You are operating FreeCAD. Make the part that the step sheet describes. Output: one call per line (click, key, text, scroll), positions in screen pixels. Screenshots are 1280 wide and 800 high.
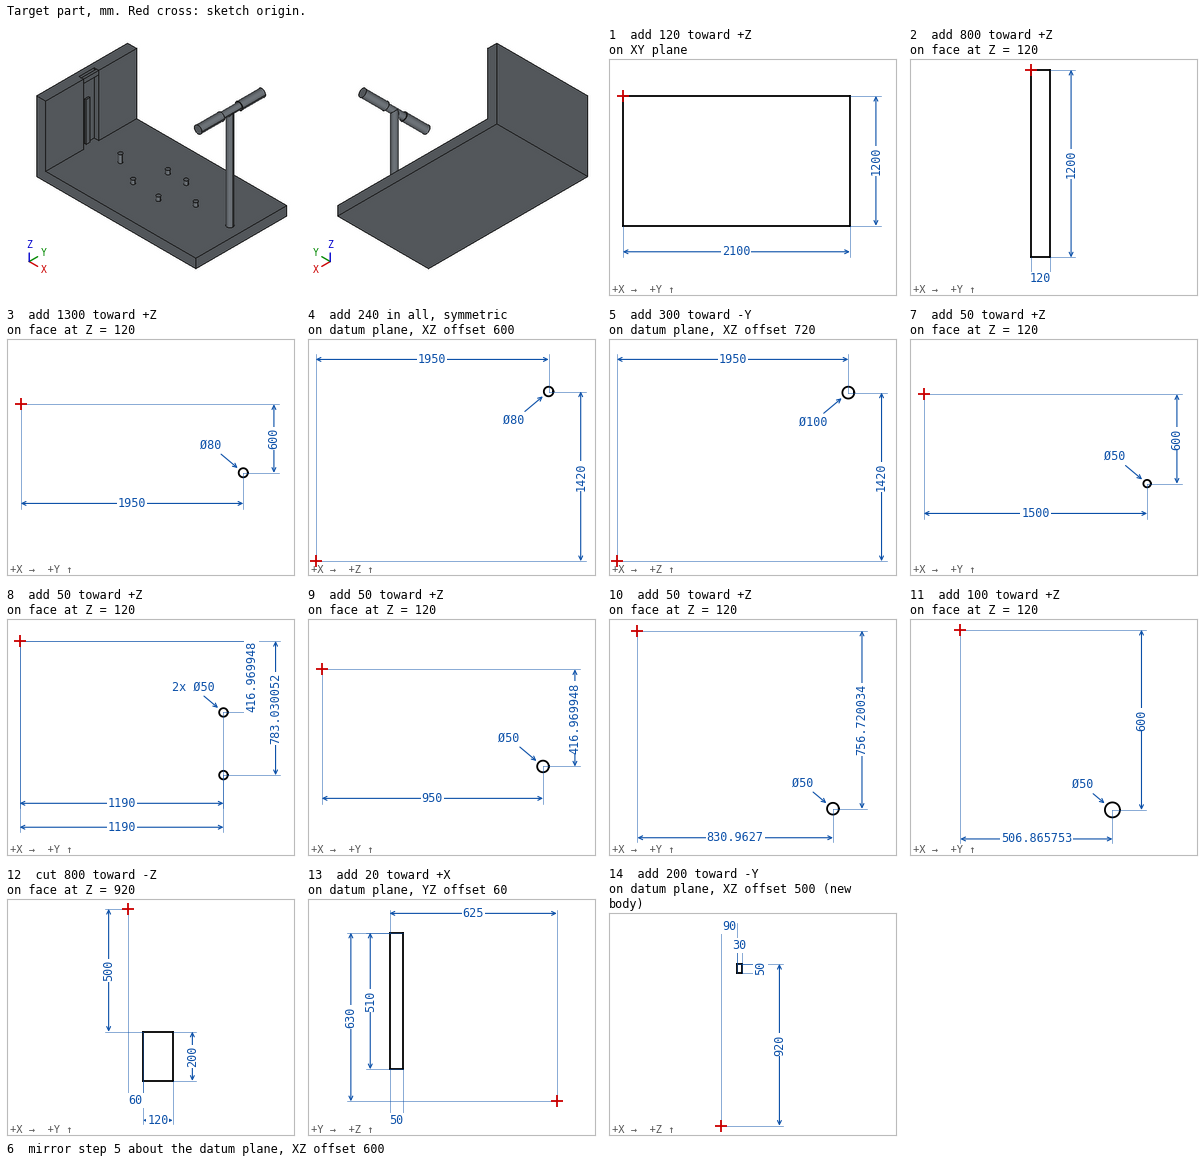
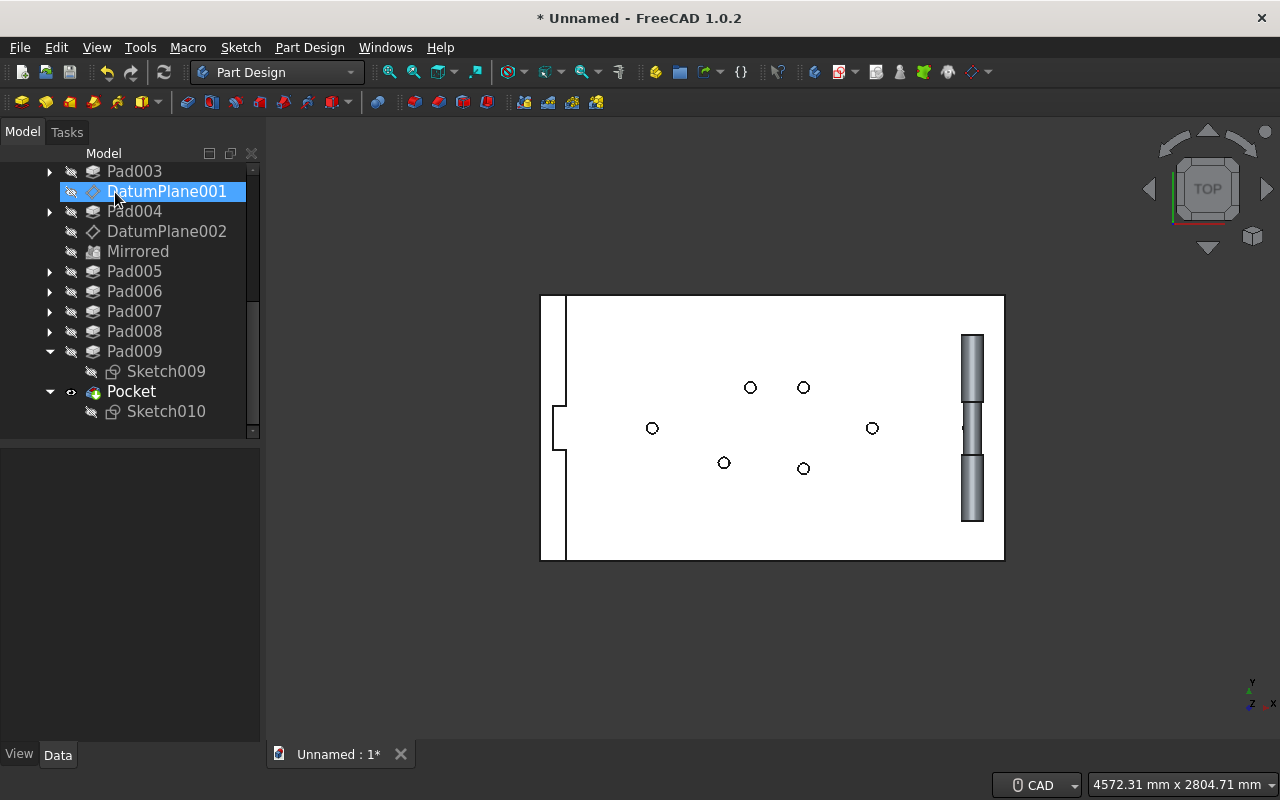
scroll(140, 287, down, 3)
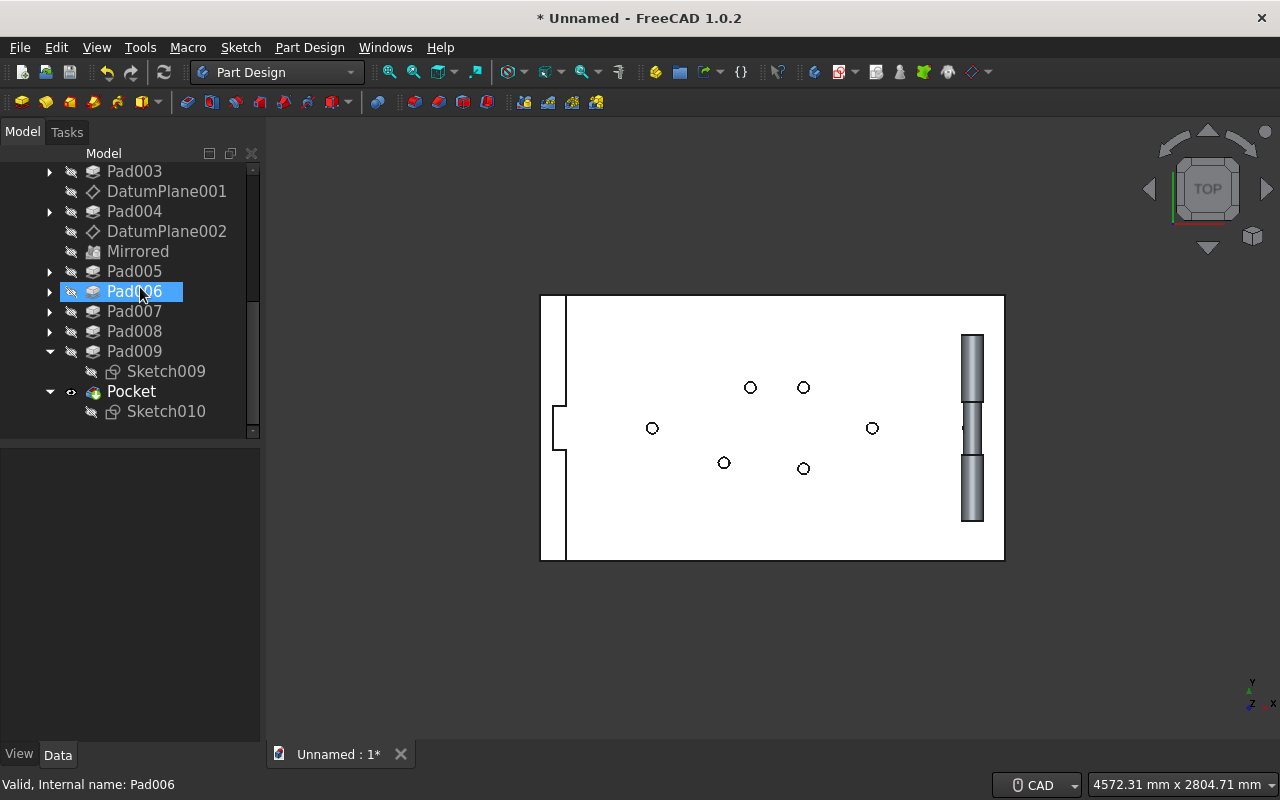
scroll(140, 287, up, 15)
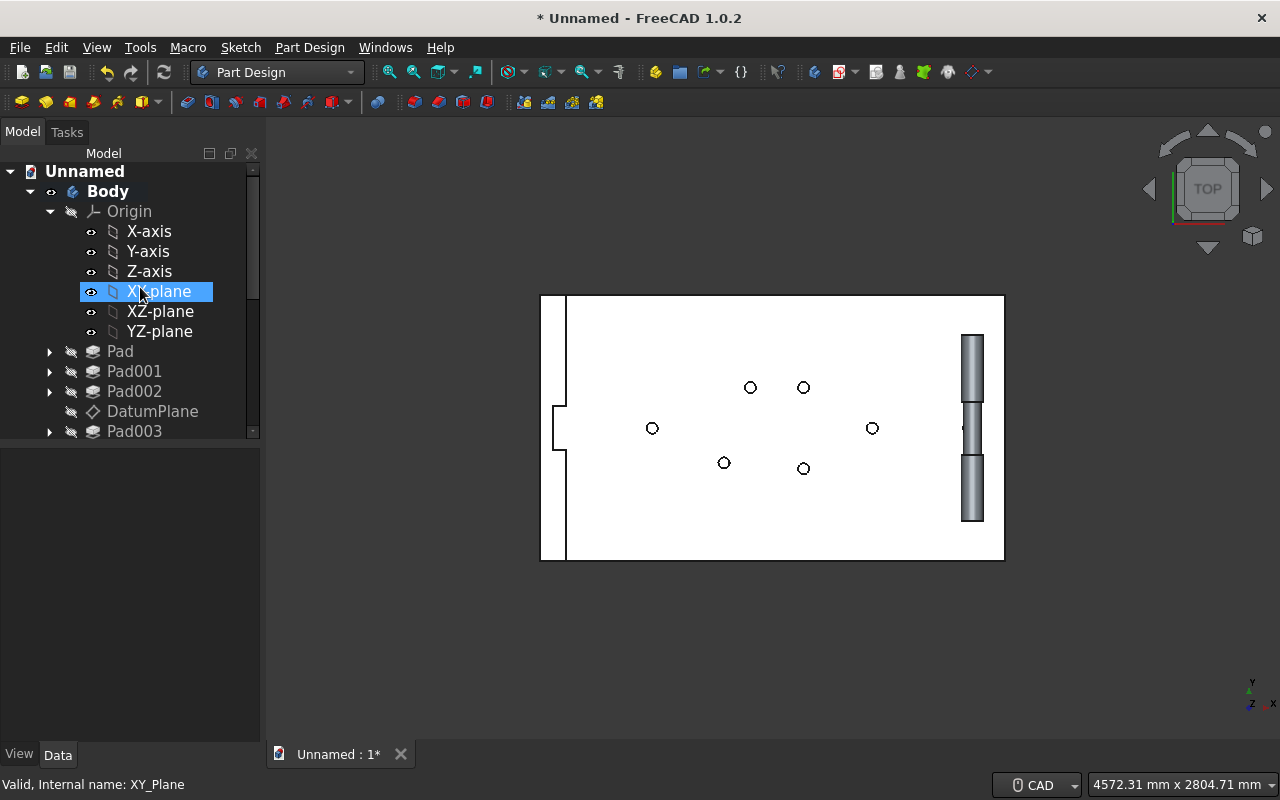
click(136, 332)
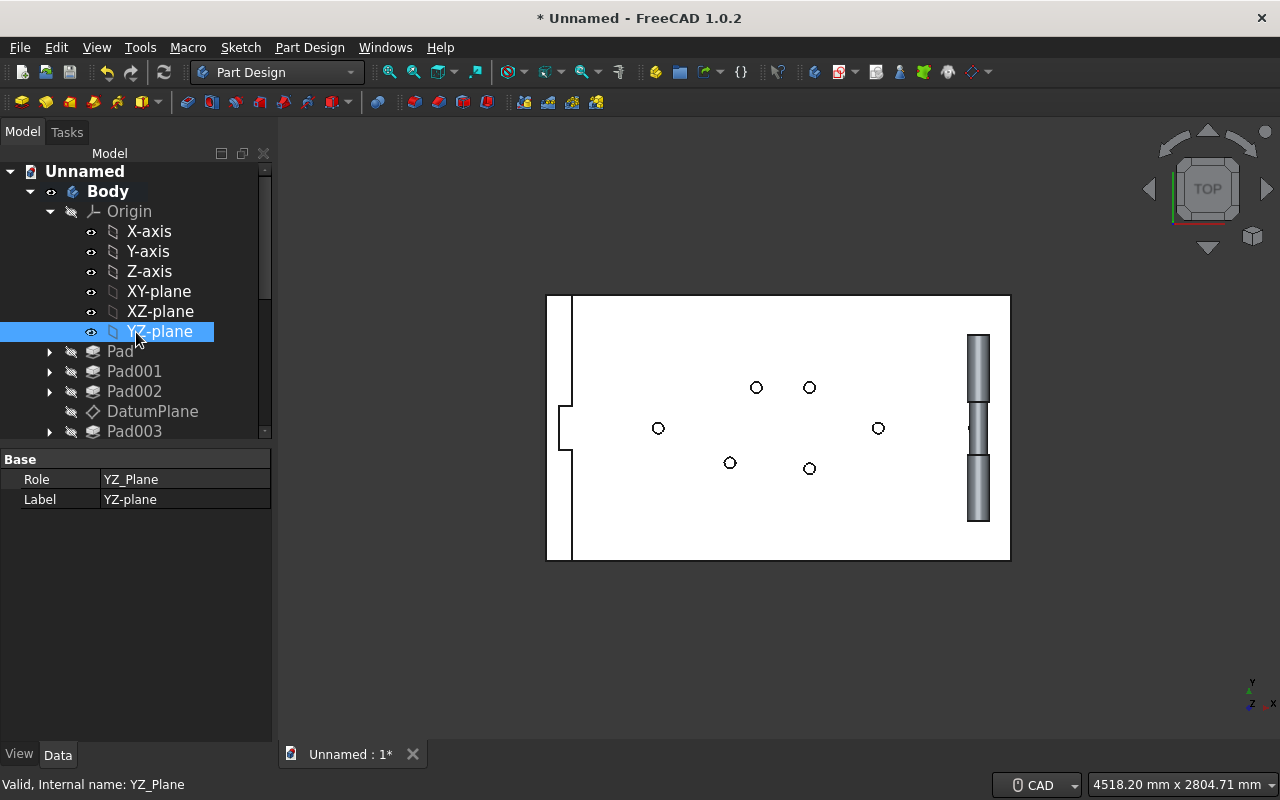
click(972, 72)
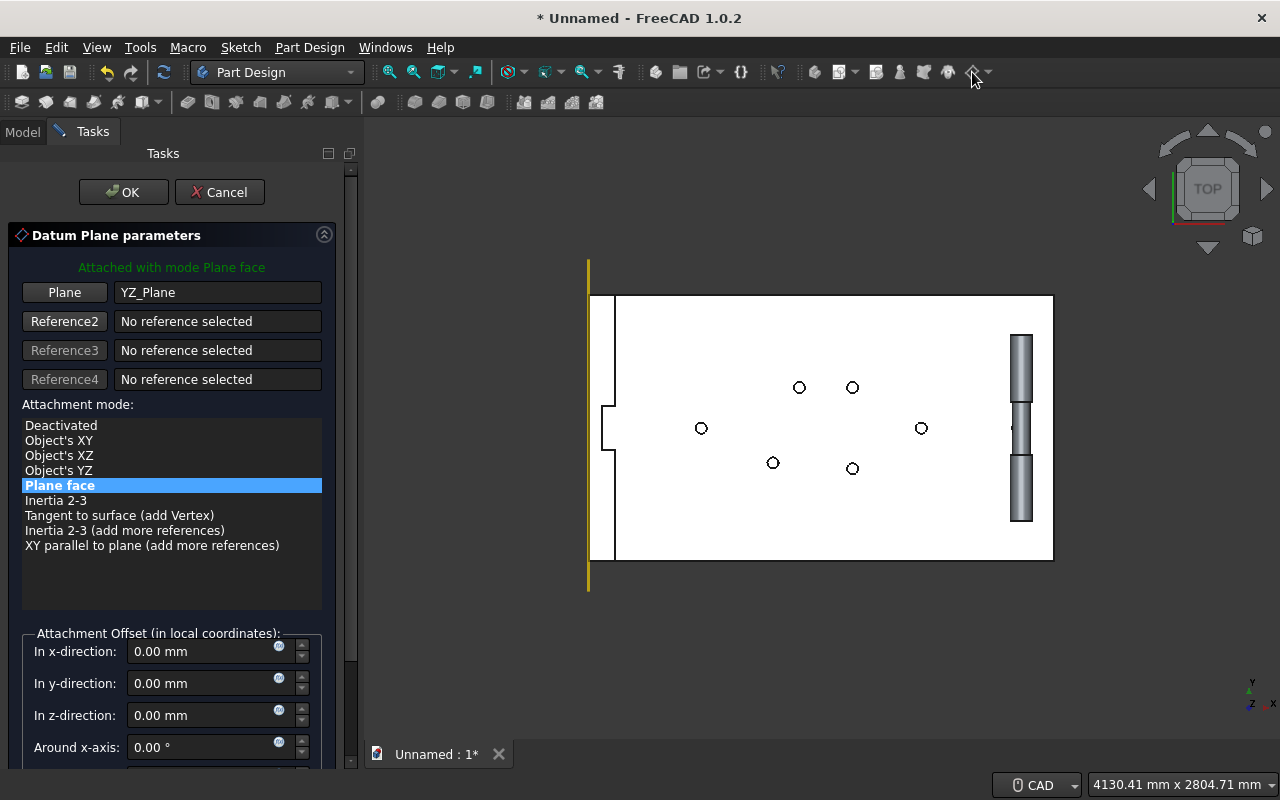
triple_click(210, 715)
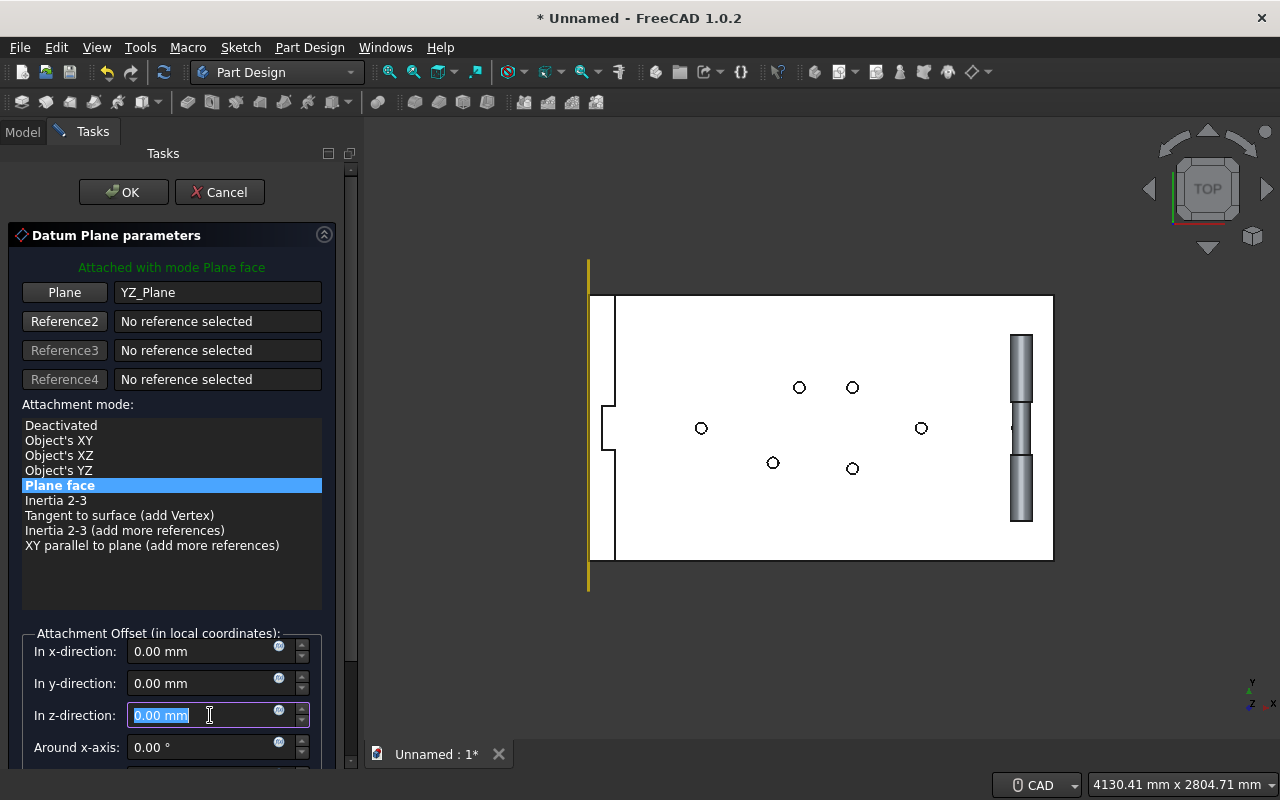
text(60)
key(Tab)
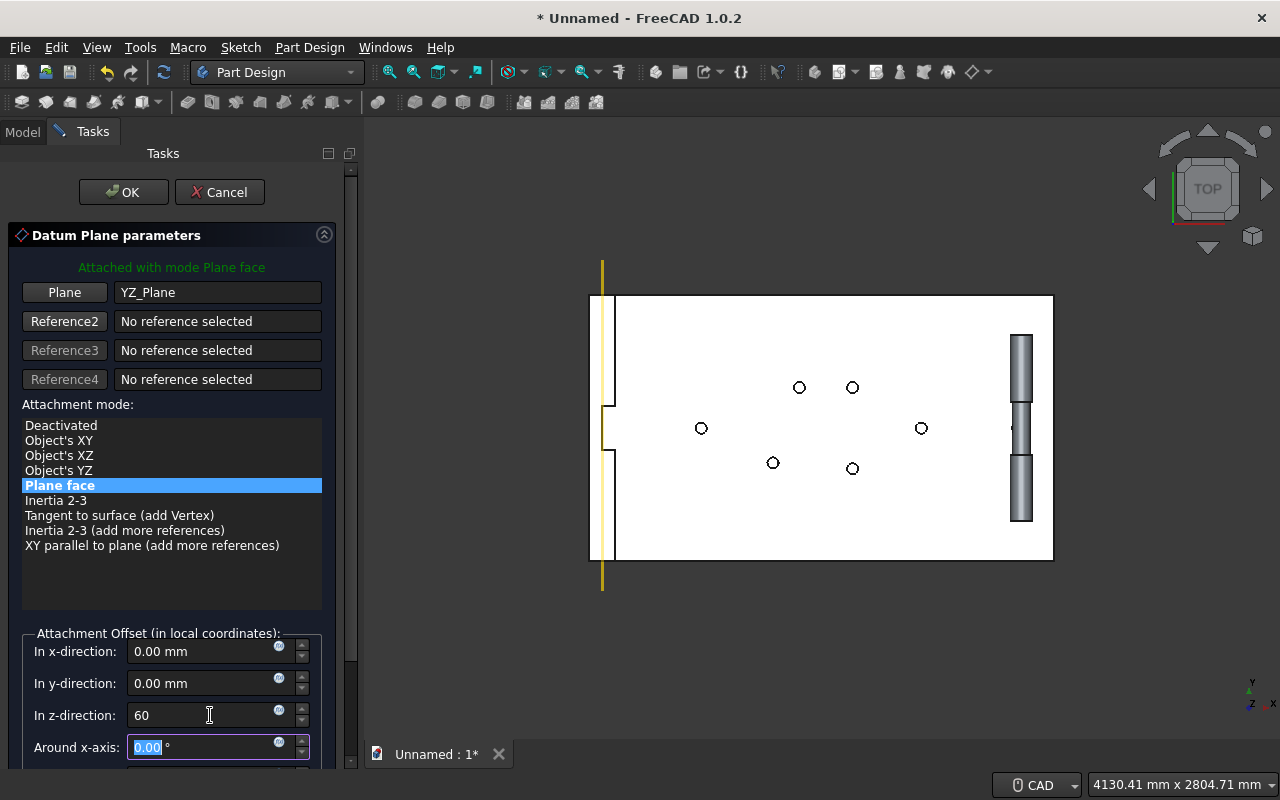
click(124, 192)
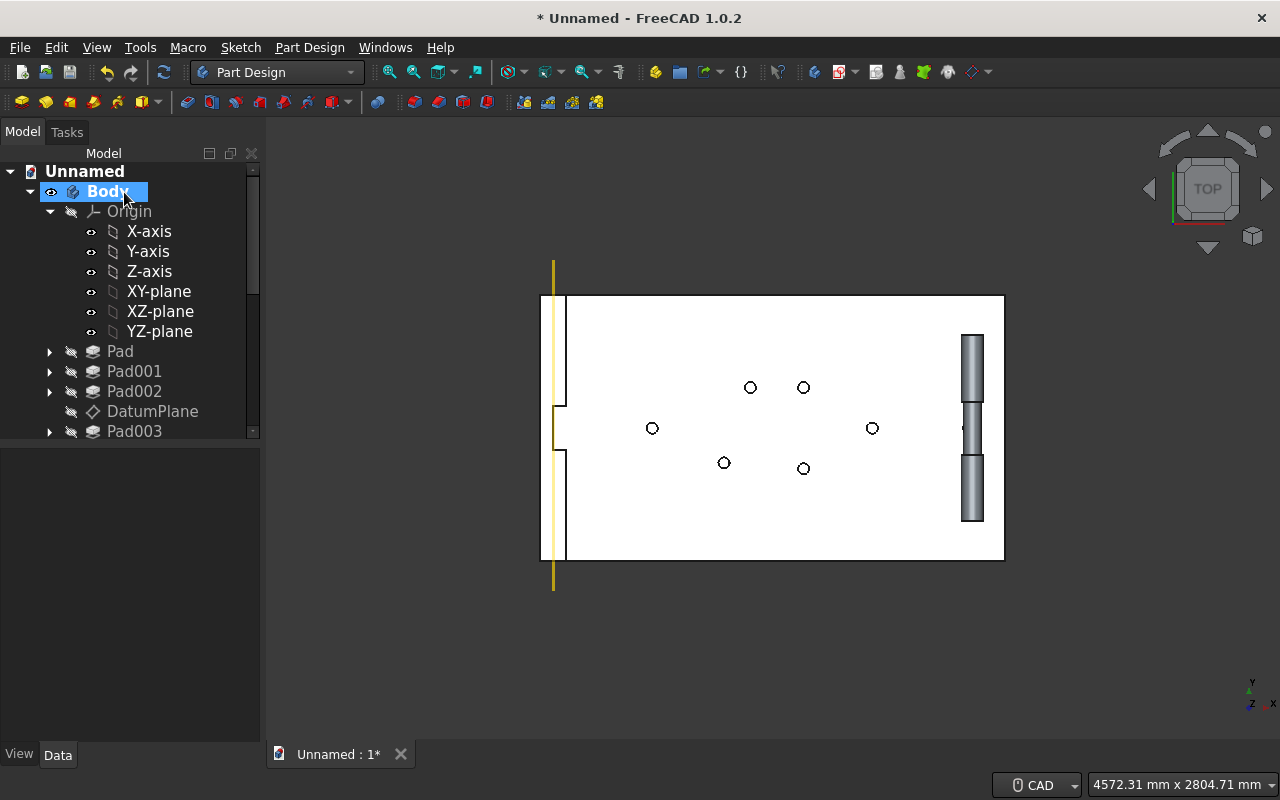
scroll(100, 307, down, 3)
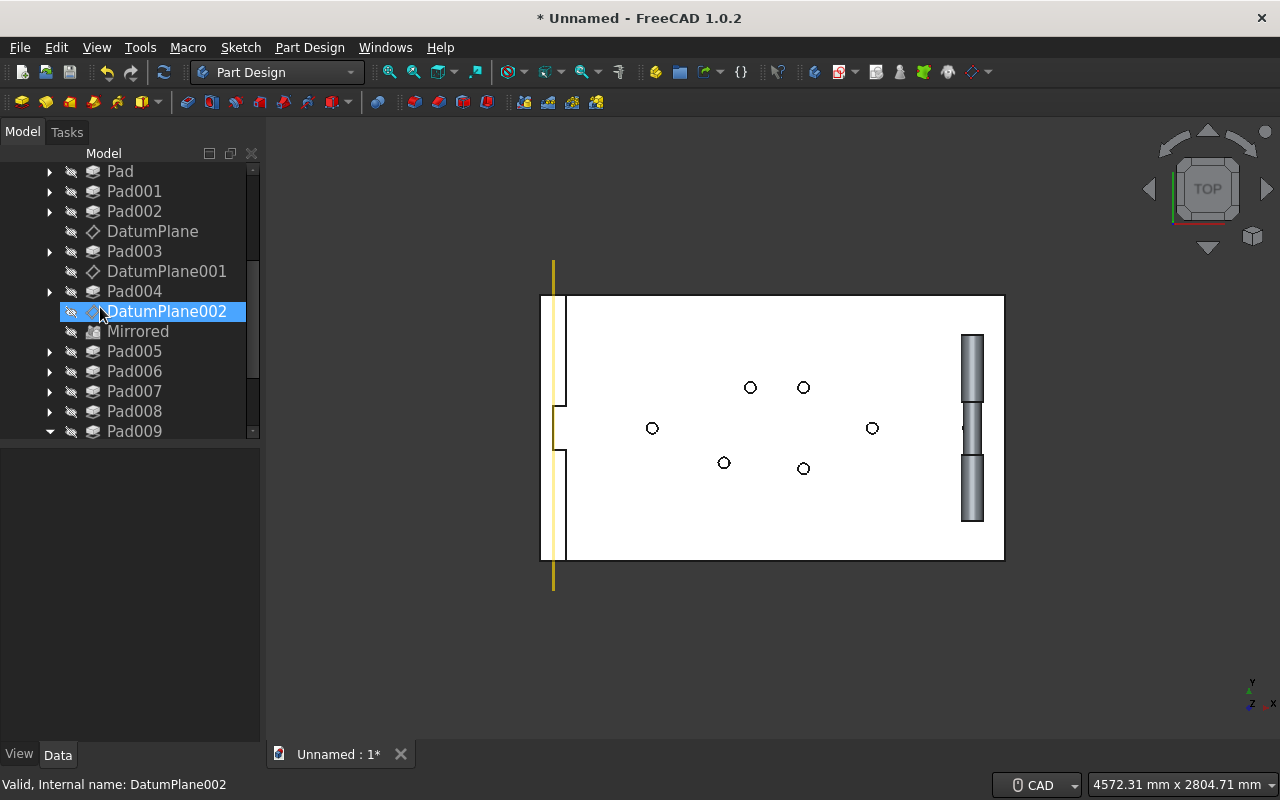
scroll(140, 307, up, 15)